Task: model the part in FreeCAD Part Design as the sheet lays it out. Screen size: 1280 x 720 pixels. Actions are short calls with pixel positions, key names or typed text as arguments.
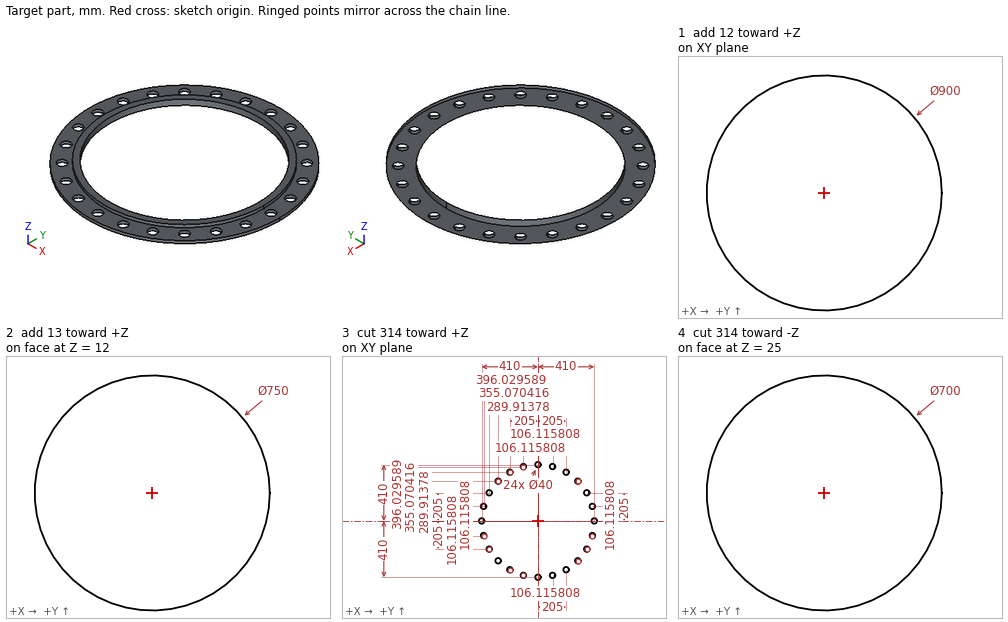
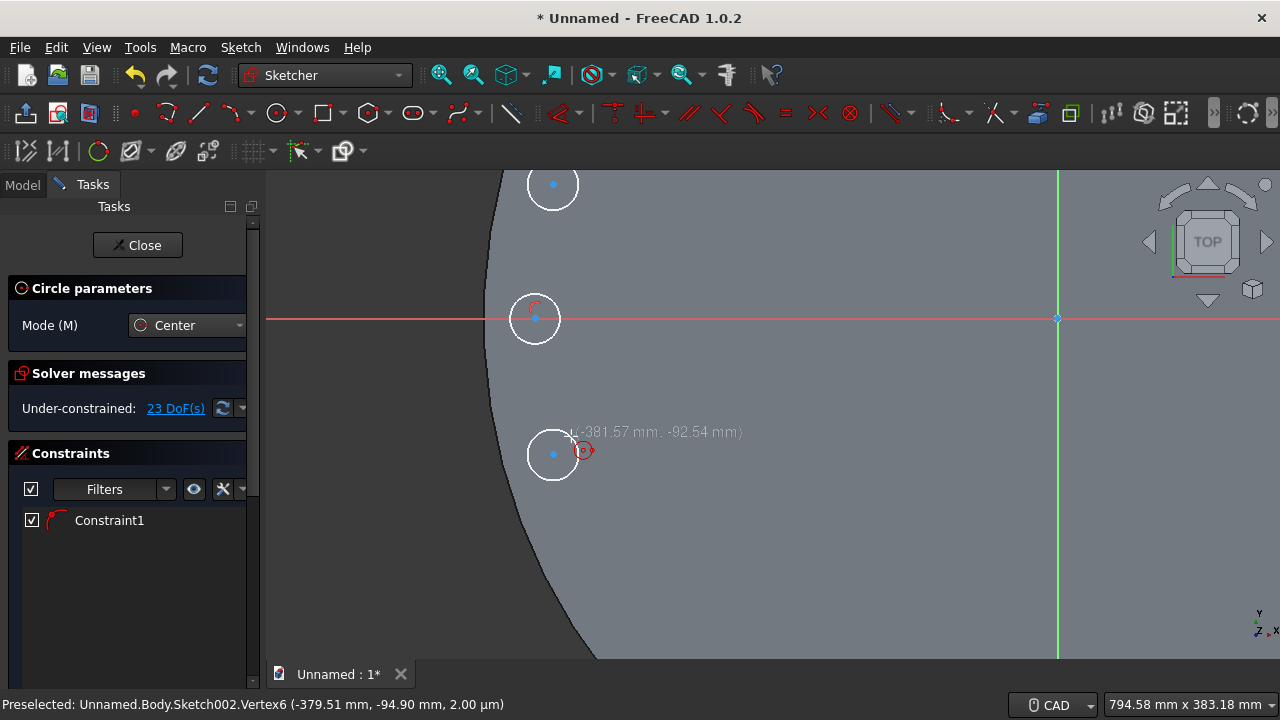
click(605, 581)
click(623, 562)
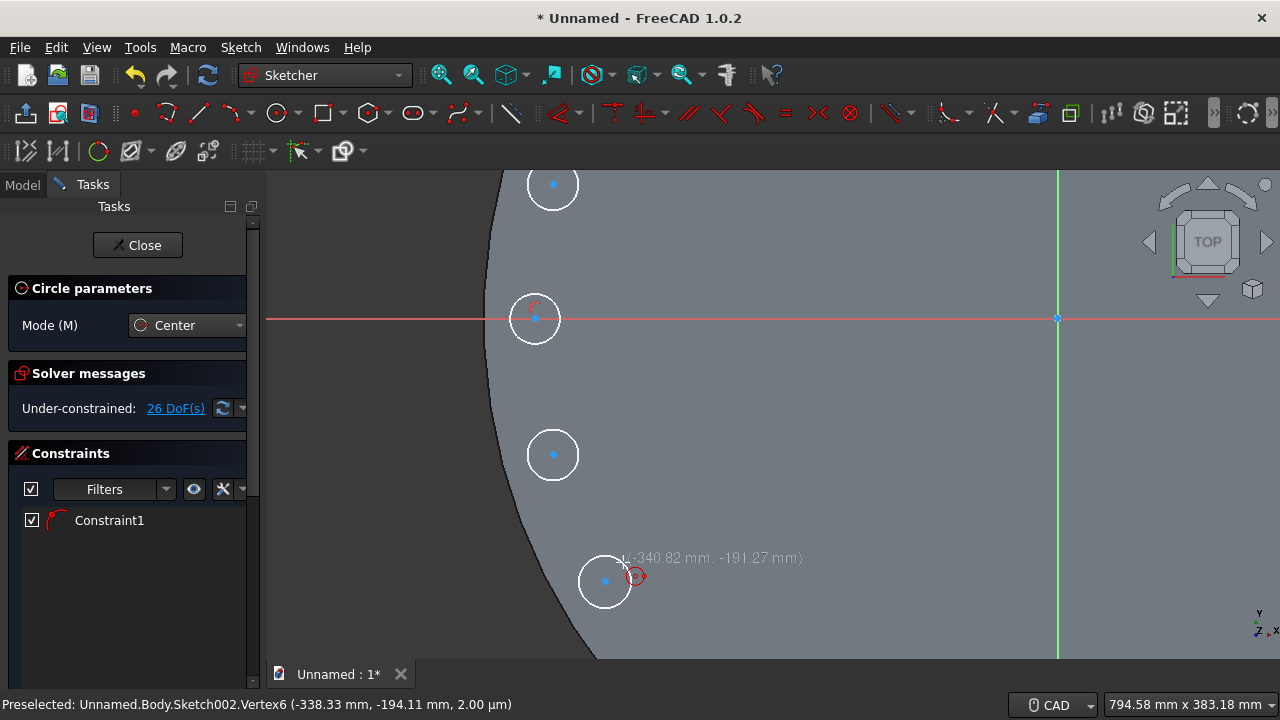
scroll(552, 456, down, 6)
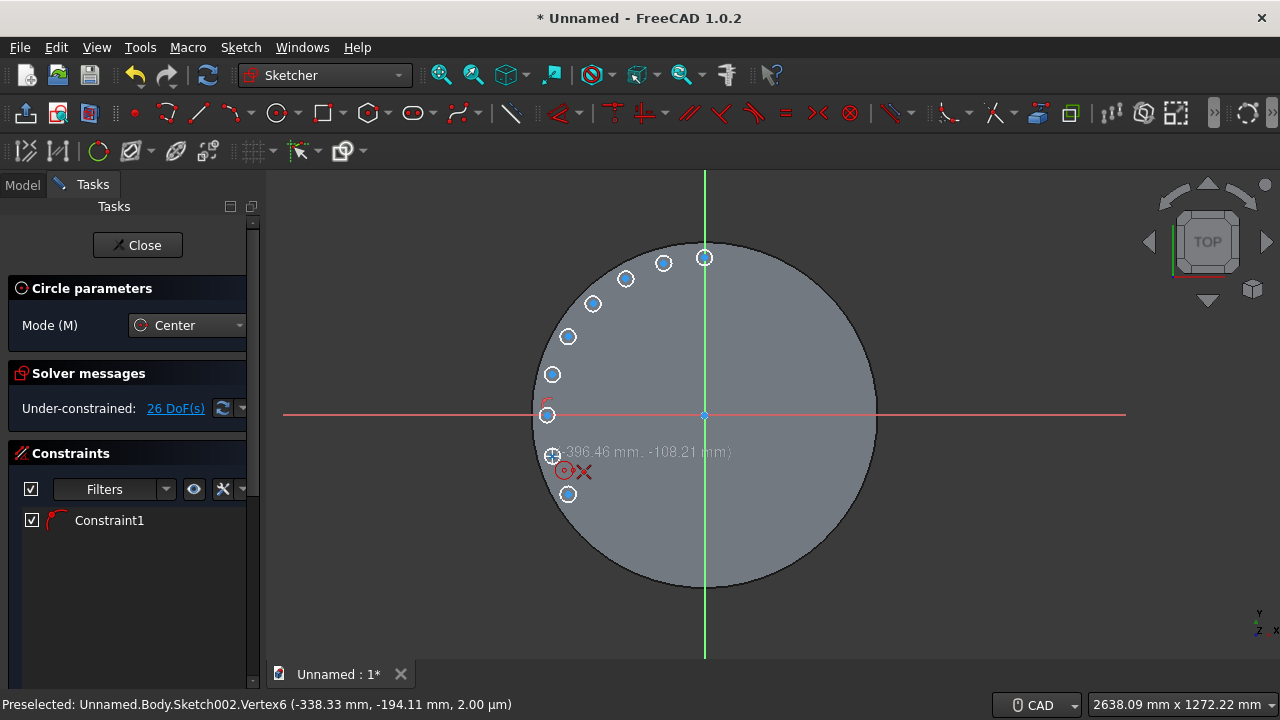
scroll(593, 527, up, 6)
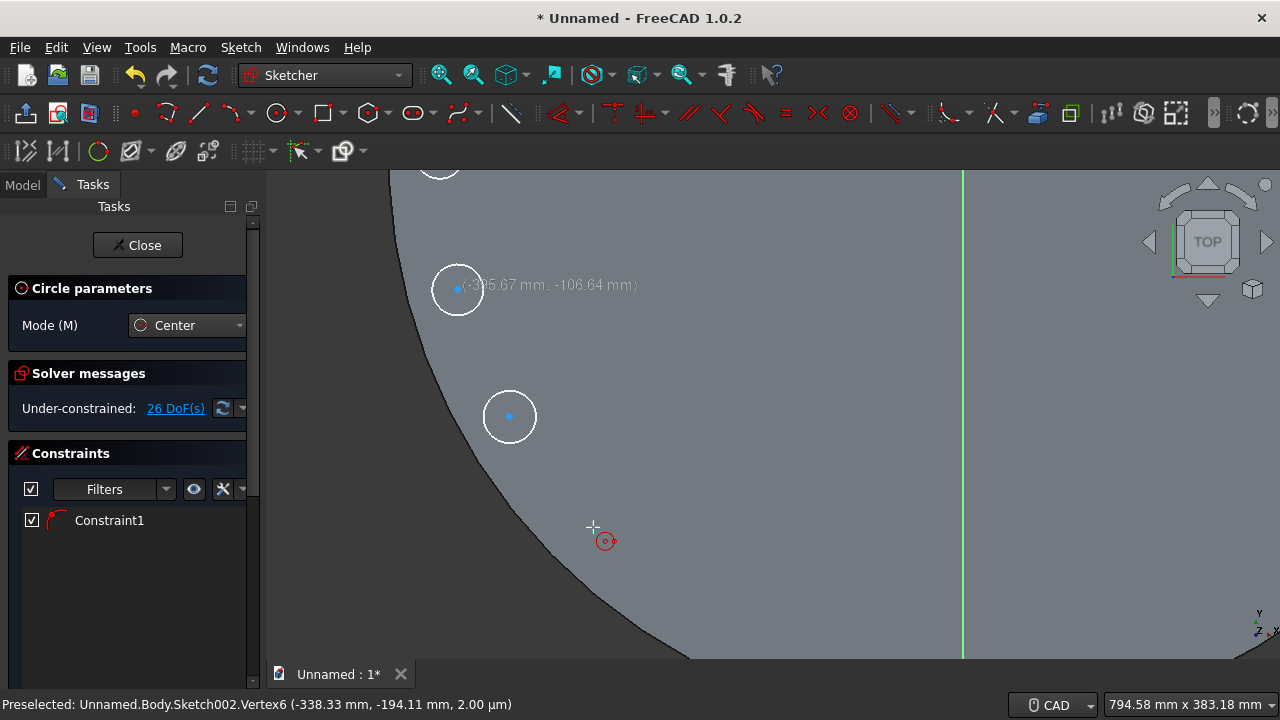
click(593, 524)
click(611, 506)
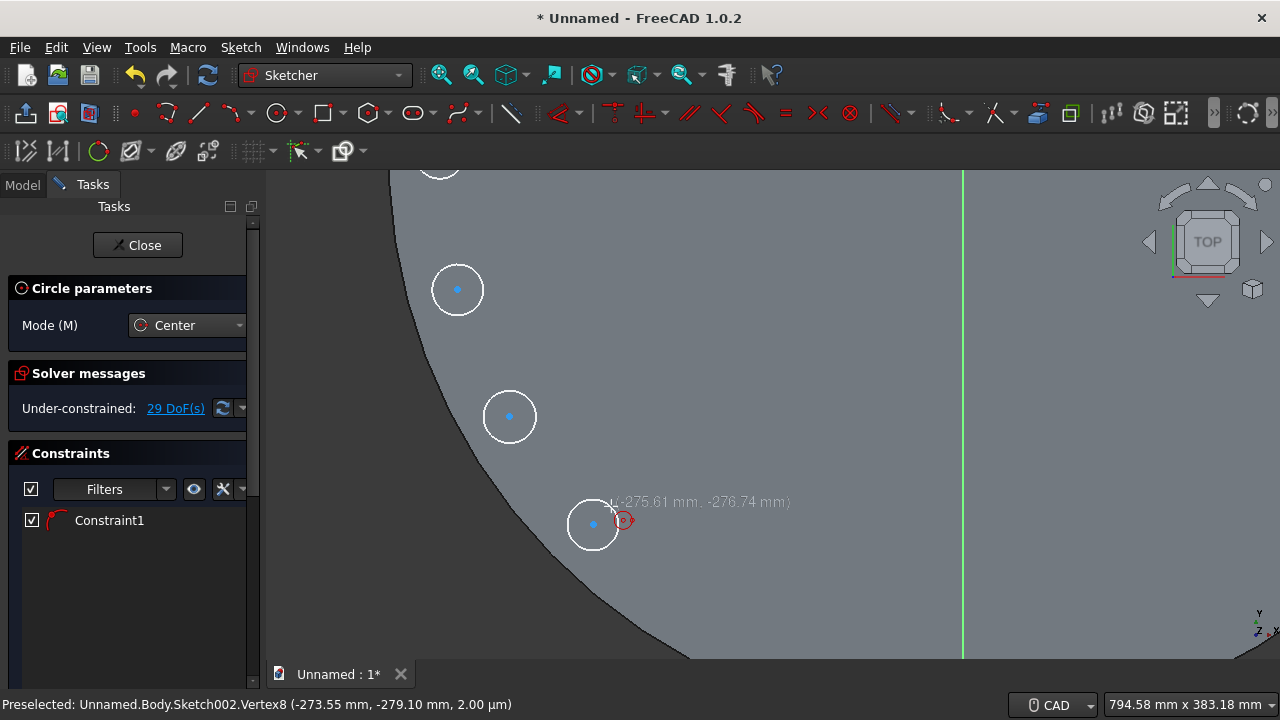
click(701, 607)
click(719, 589)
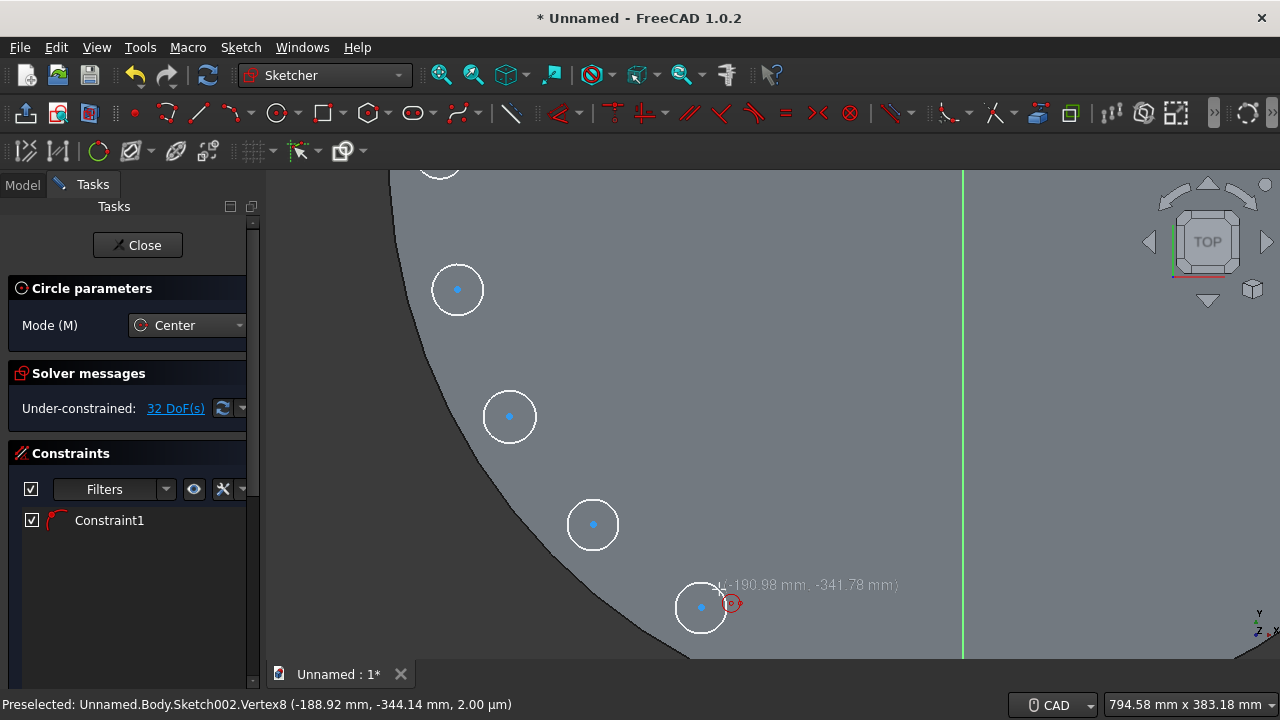
scroll(593, 527, down, 6)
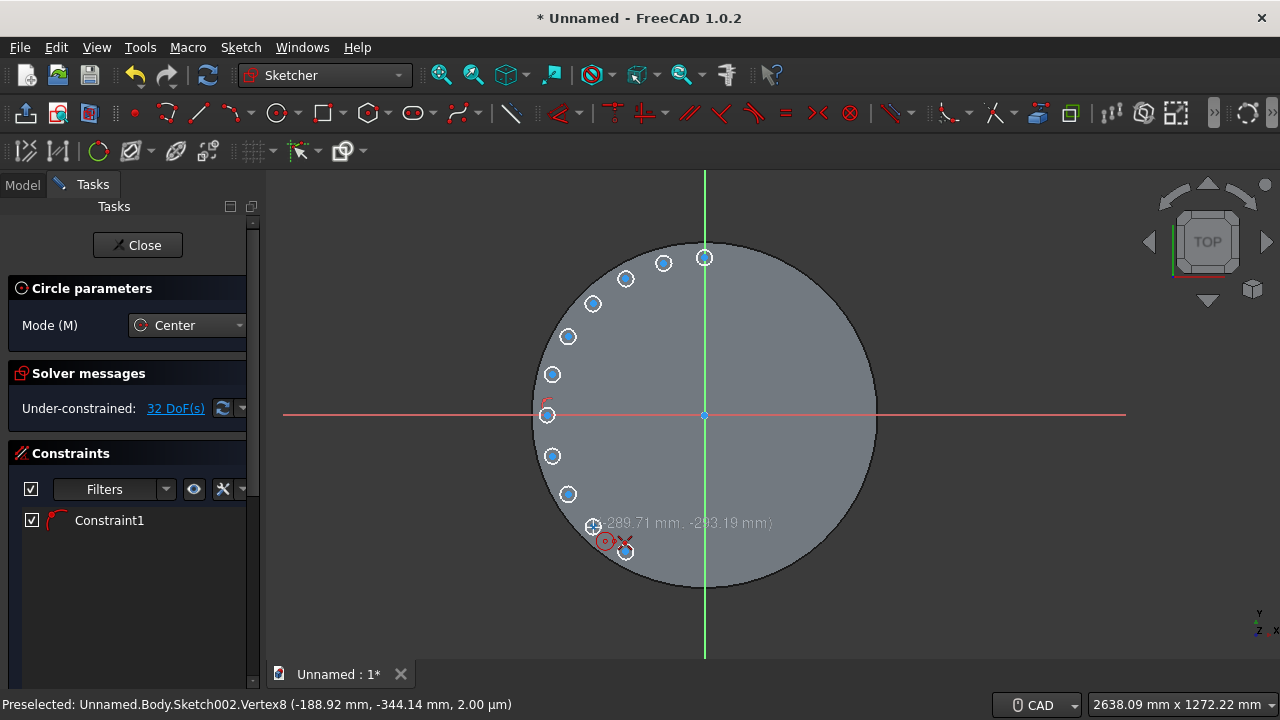
scroll(664, 567, up, 6)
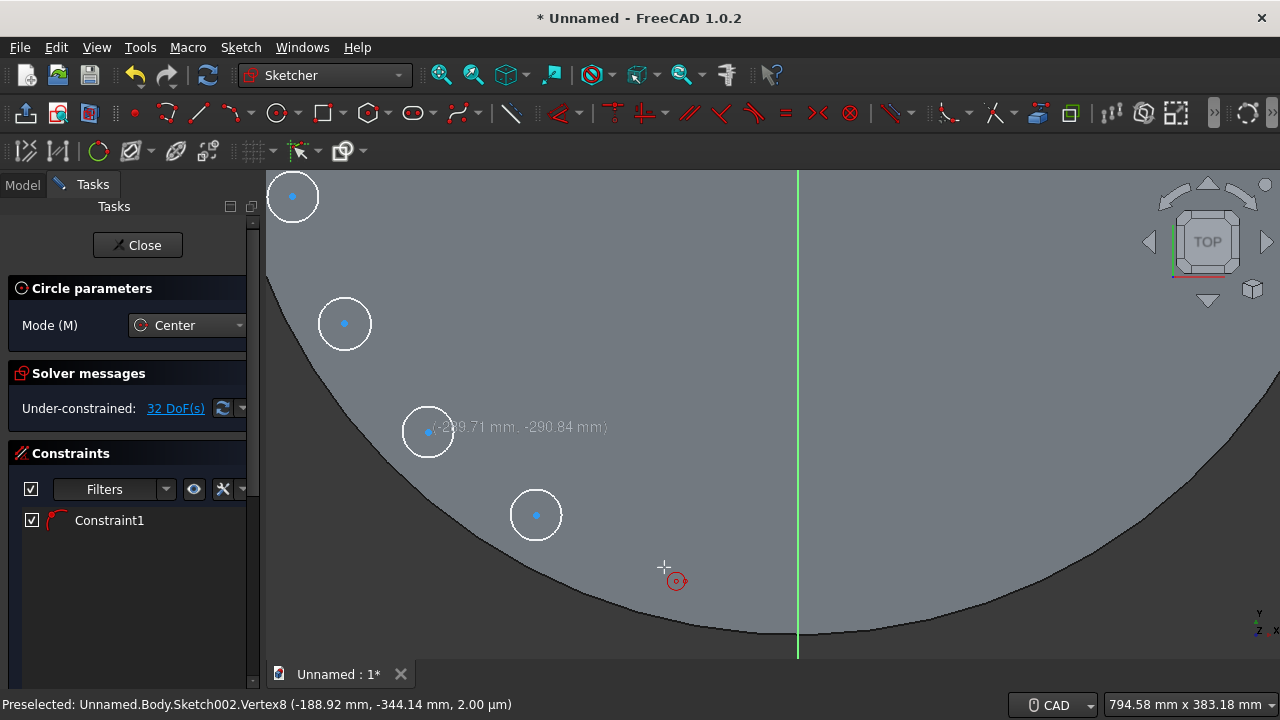
click(662, 566)
click(680, 548)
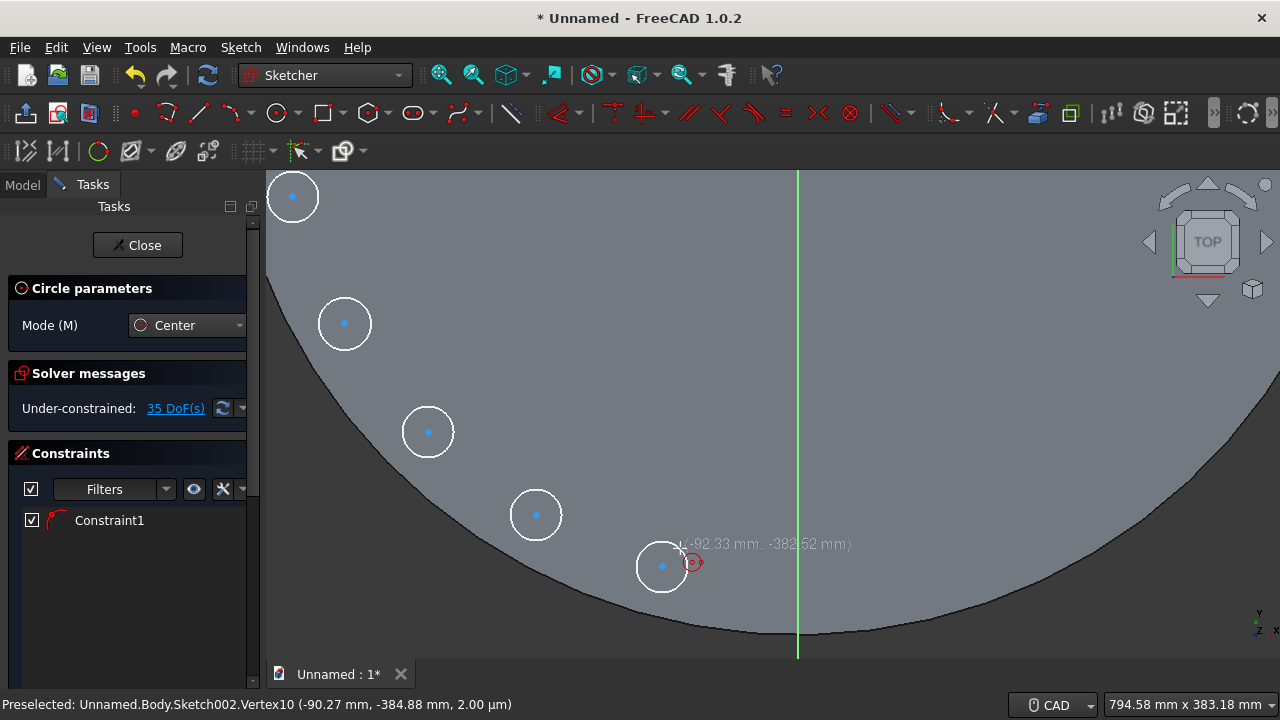
click(798, 584)
click(816, 566)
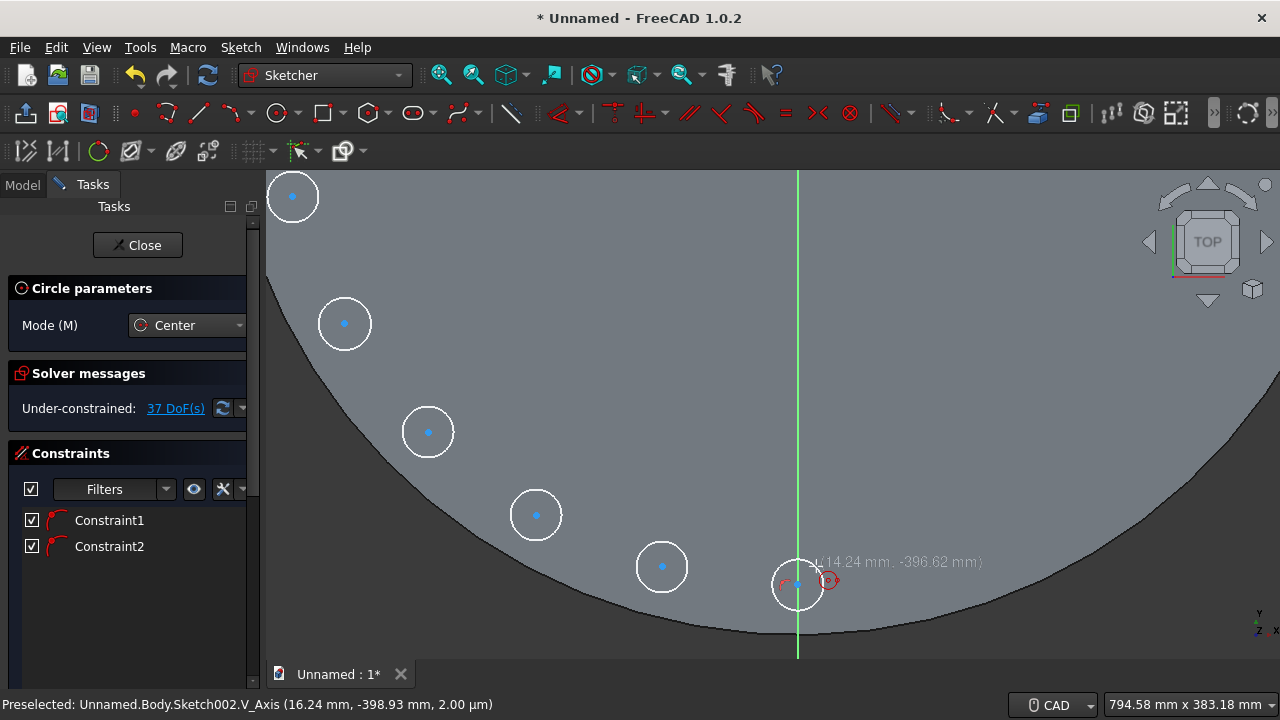
click(933, 566)
click(951, 548)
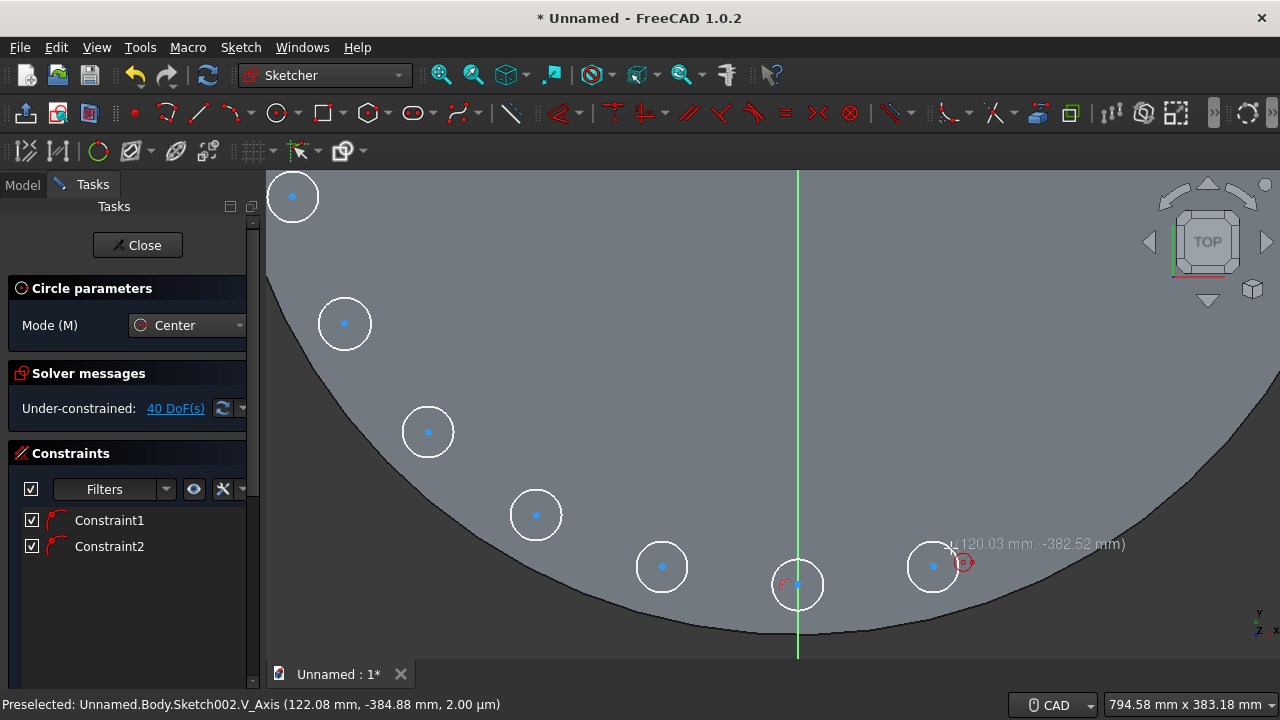
click(1059, 514)
click(1077, 496)